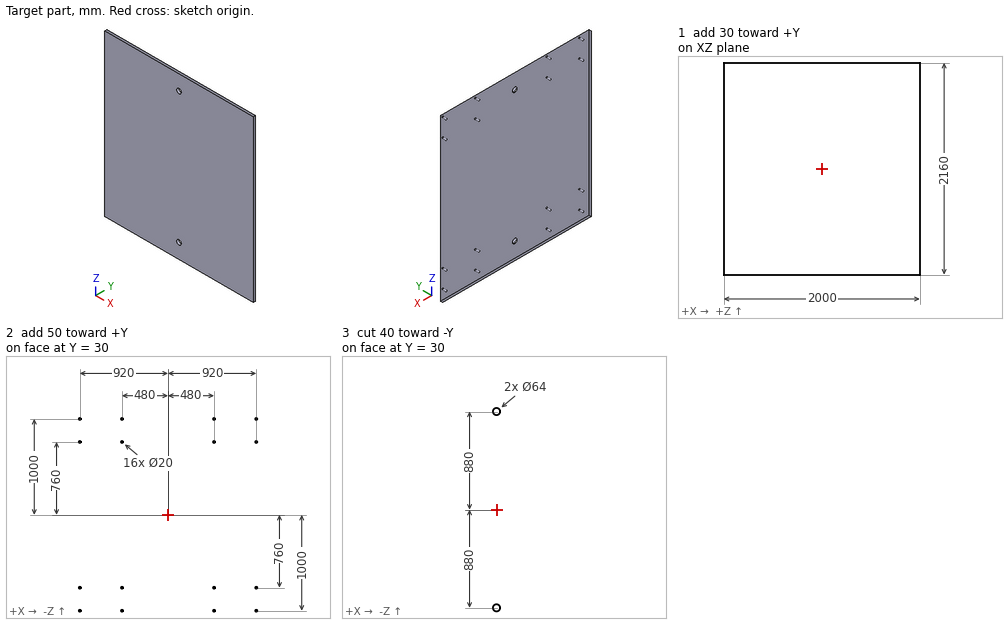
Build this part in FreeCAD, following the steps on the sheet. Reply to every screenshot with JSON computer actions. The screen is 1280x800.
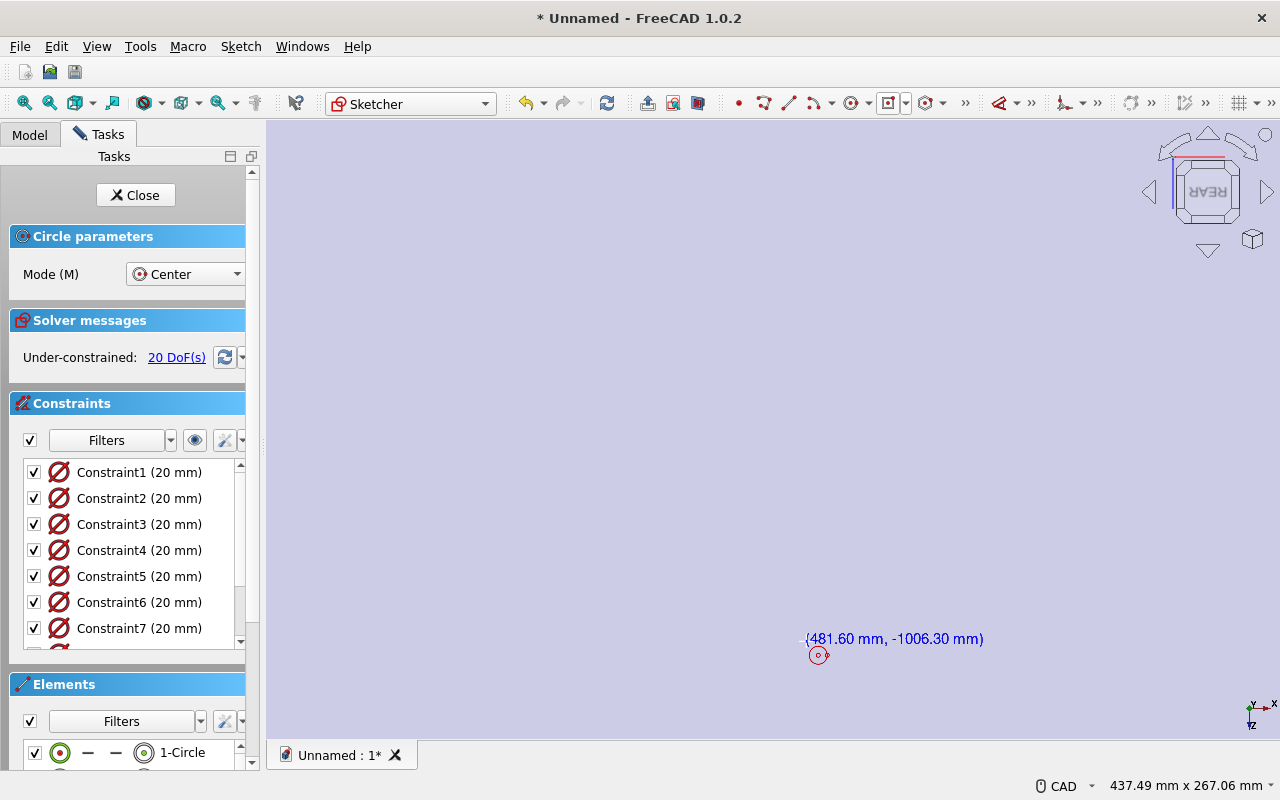
{"action": "scroll", "coordinate": [806, 641], "scroll_direction": "down", "scroll_amount": 12}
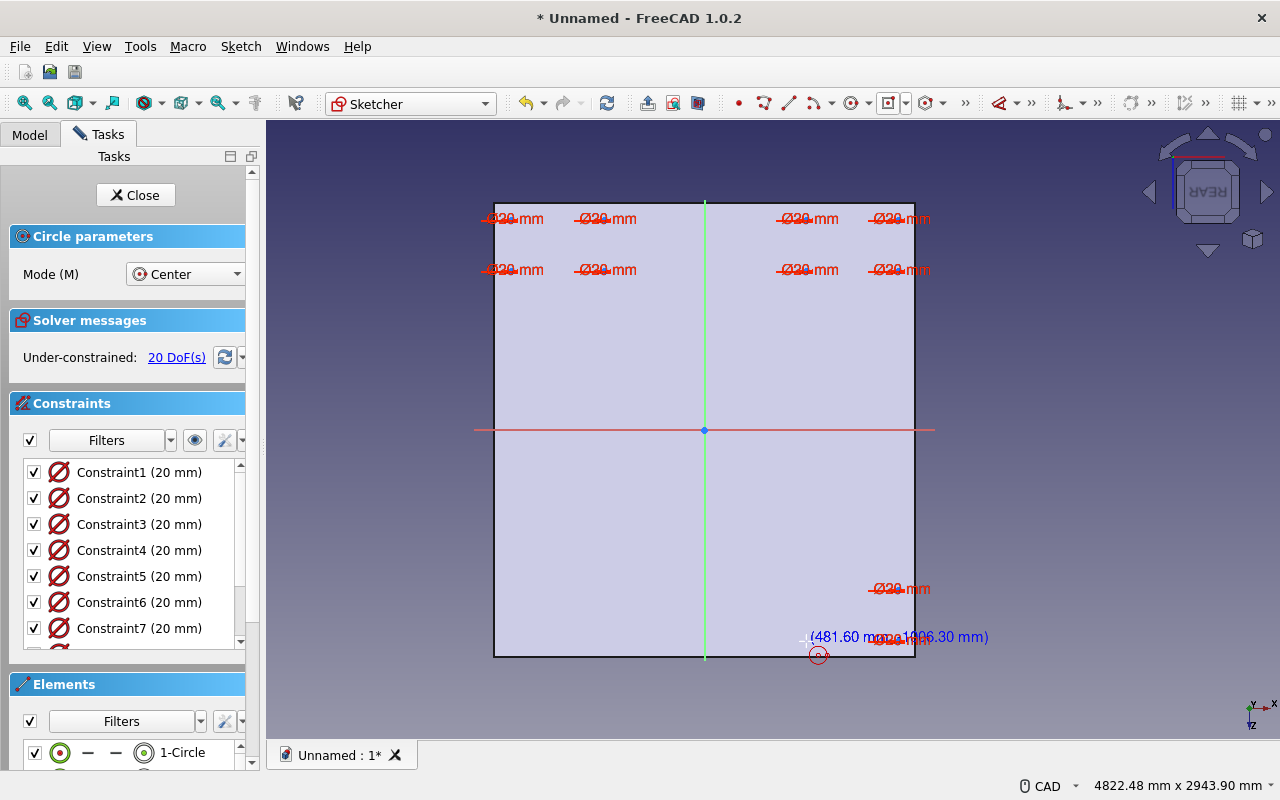
{"action": "left_click", "coordinate": [806, 641]}
{"action": "mouse_move", "coordinate": [807, 639]}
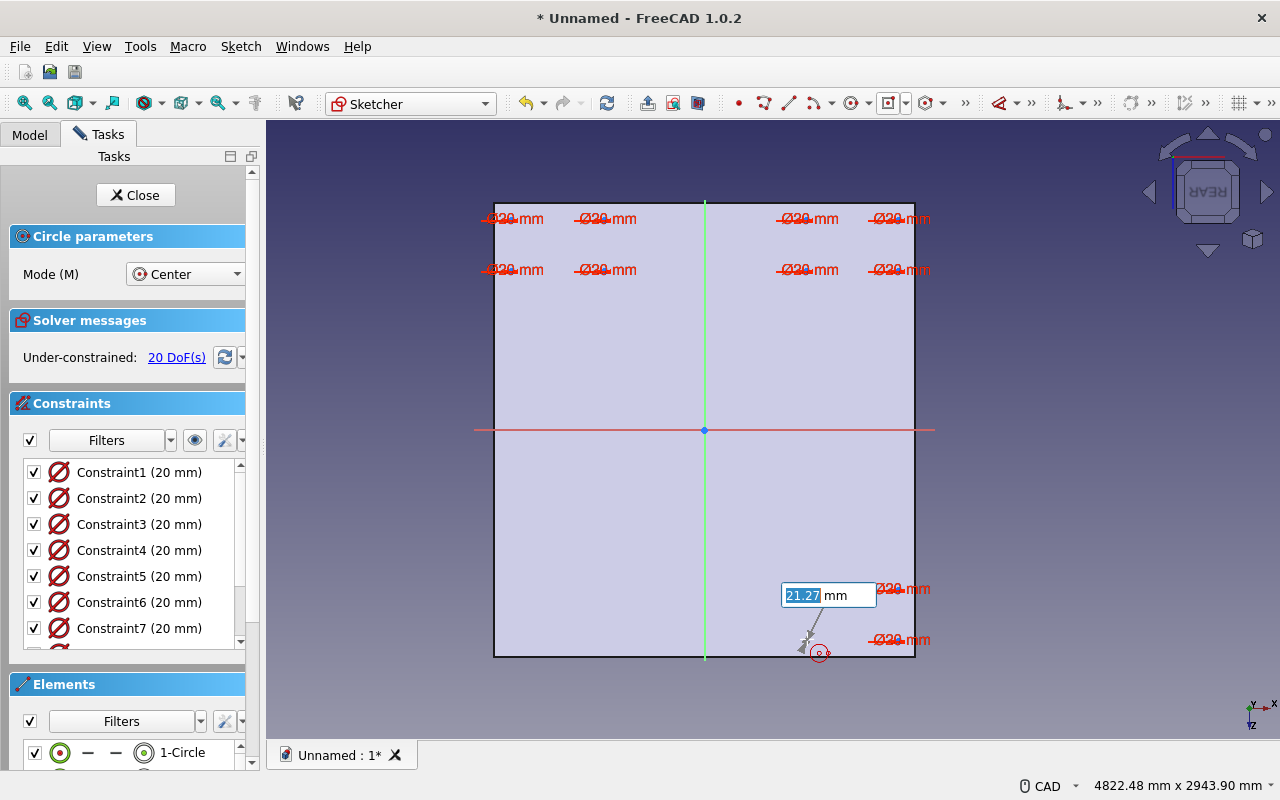
{"action": "type", "text": "20"}
{"action": "key", "text": "Return"}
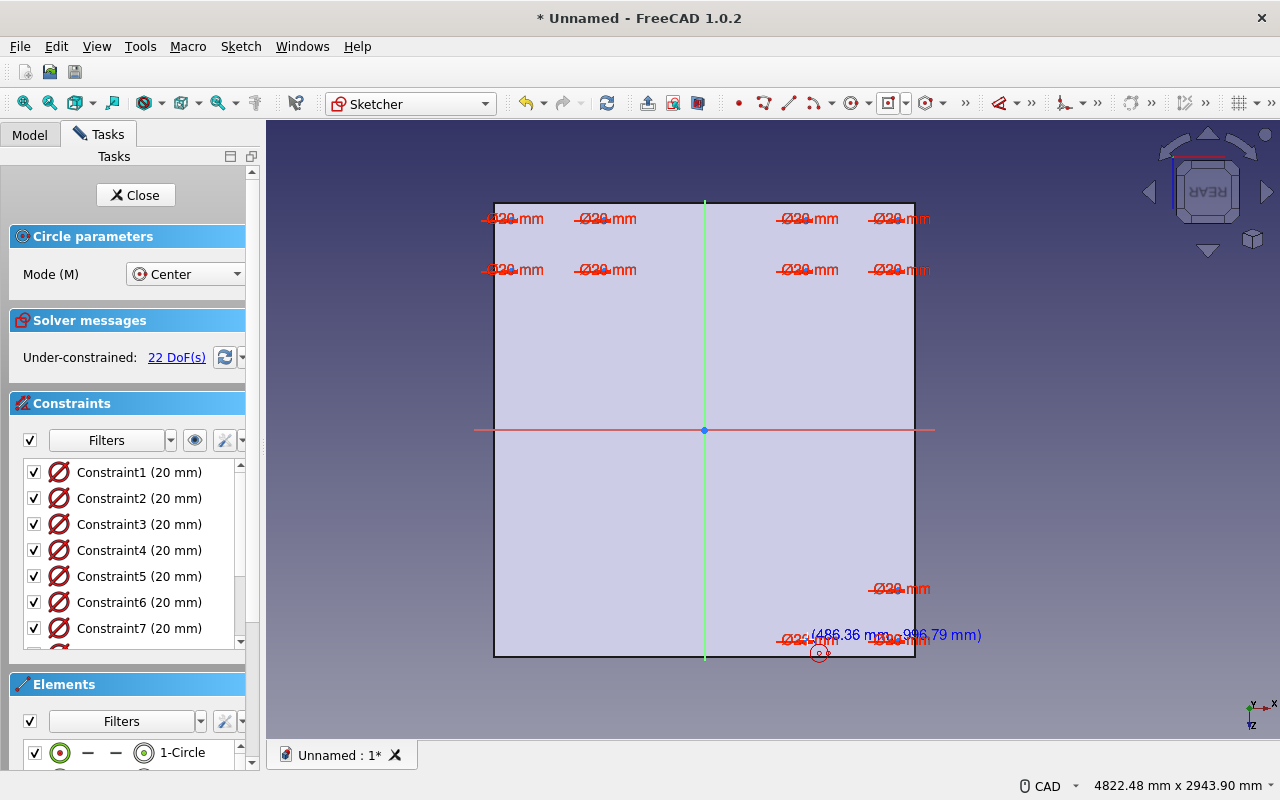
{"action": "scroll", "coordinate": [806, 590], "scroll_direction": "up", "scroll_amount": 12}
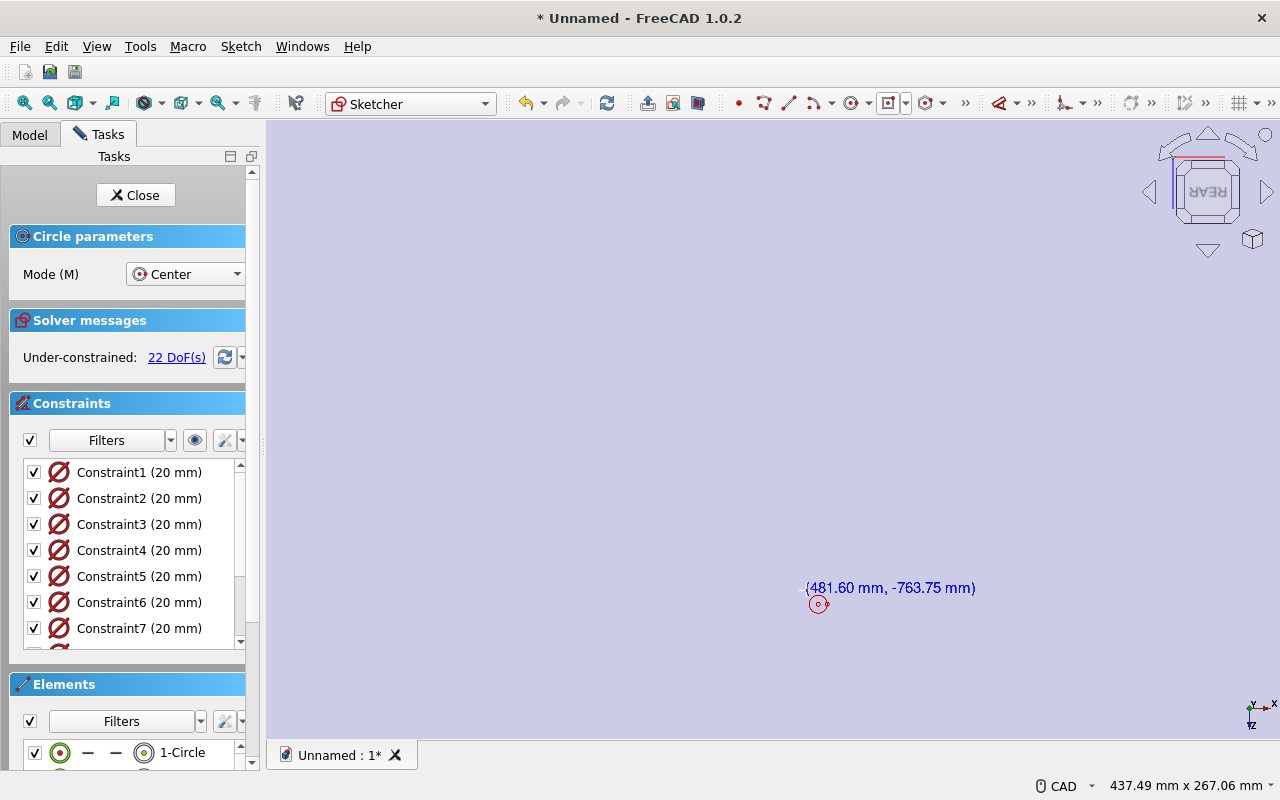
{"action": "scroll", "coordinate": [806, 590], "scroll_direction": "down", "scroll_amount": 12}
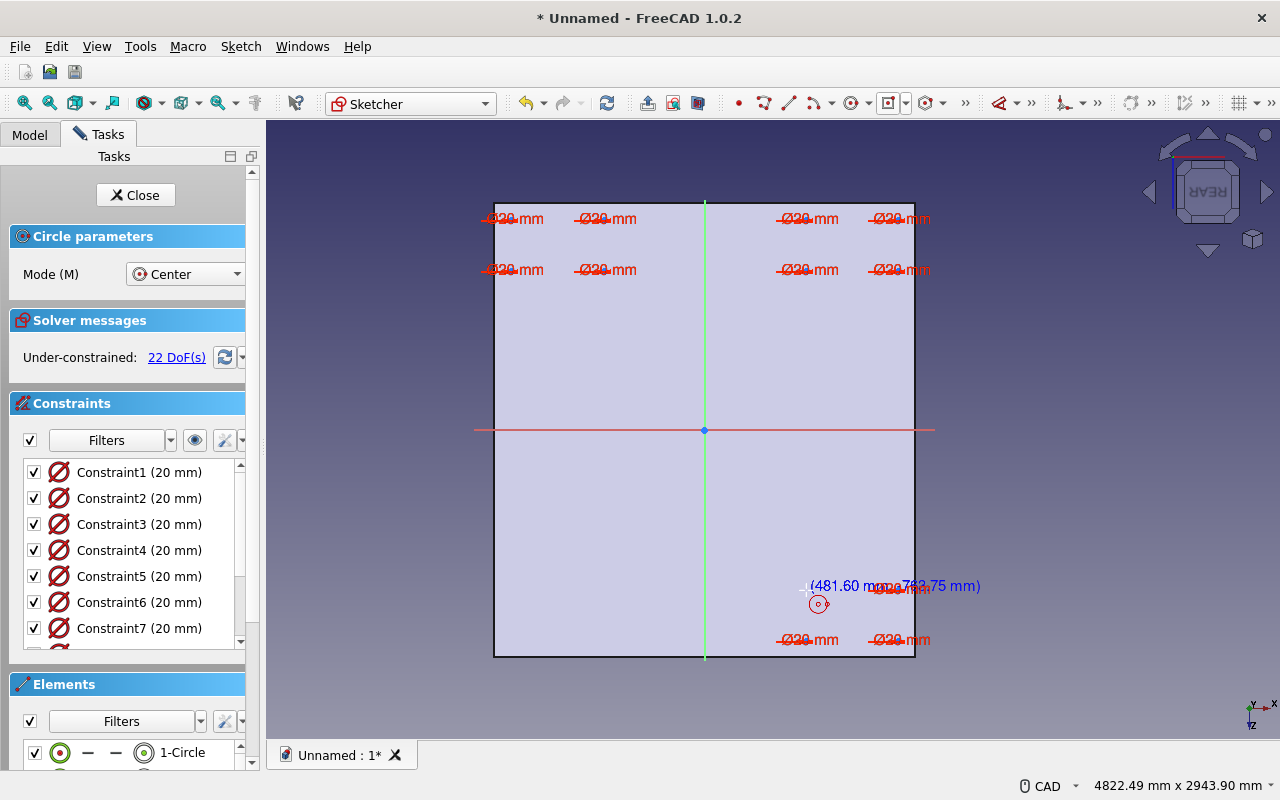
{"action": "left_click", "coordinate": [806, 590]}
{"action": "mouse_move", "coordinate": [807, 589]}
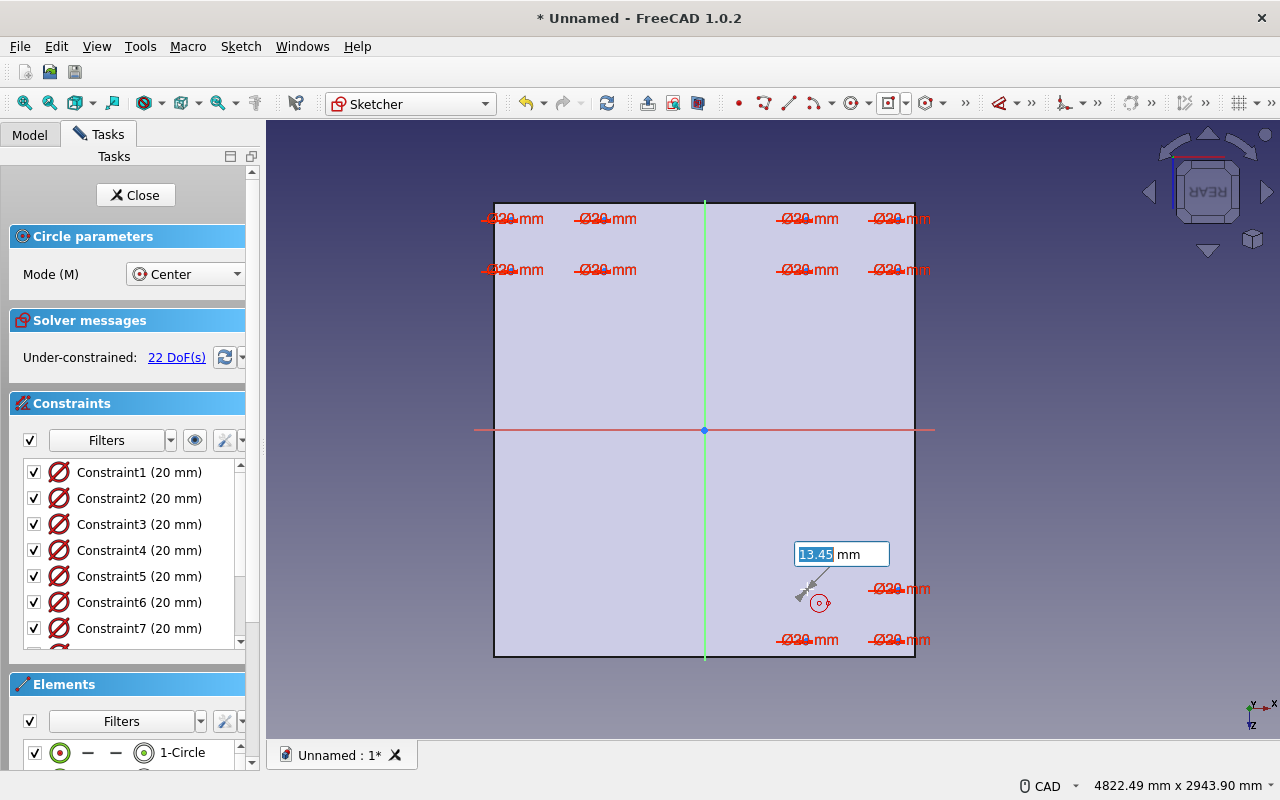
{"action": "type", "text": "20"}
{"action": "key", "text": "Return"}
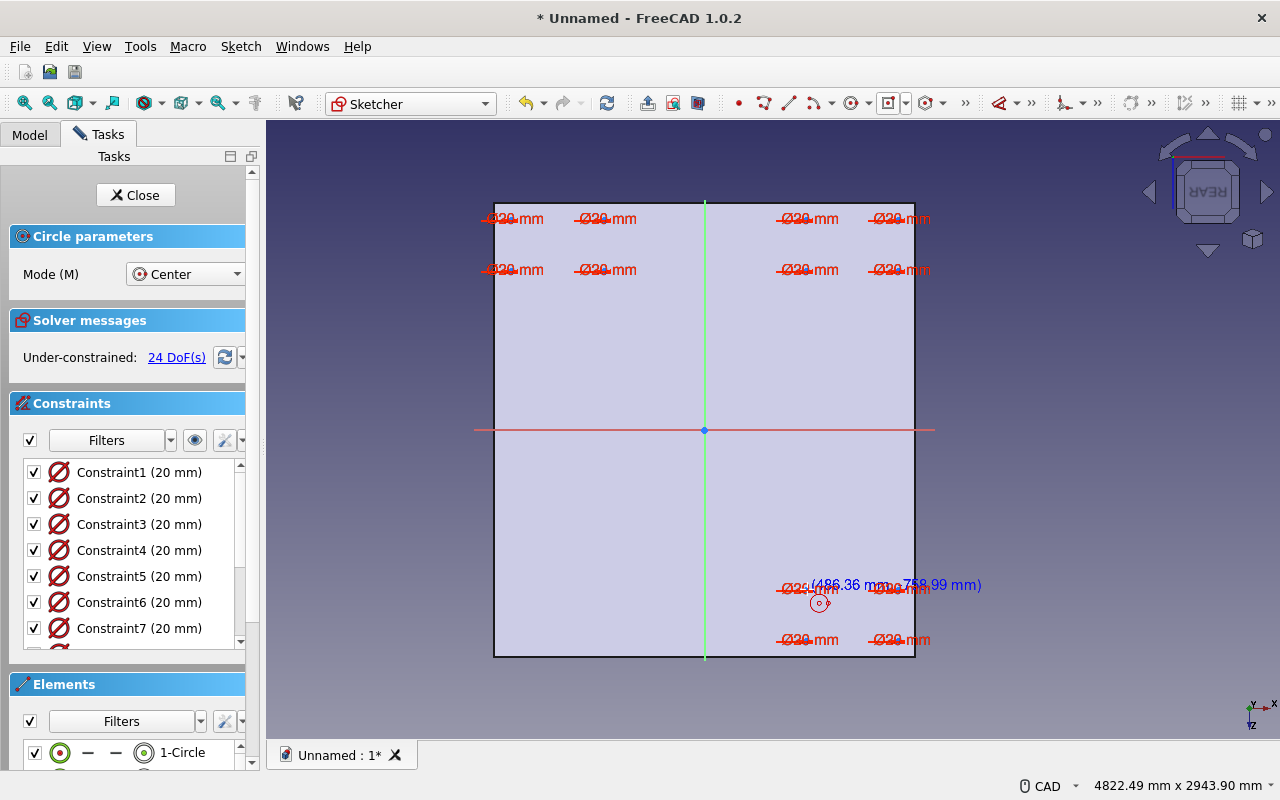
{"action": "scroll", "coordinate": [604, 590], "scroll_direction": "up", "scroll_amount": 12}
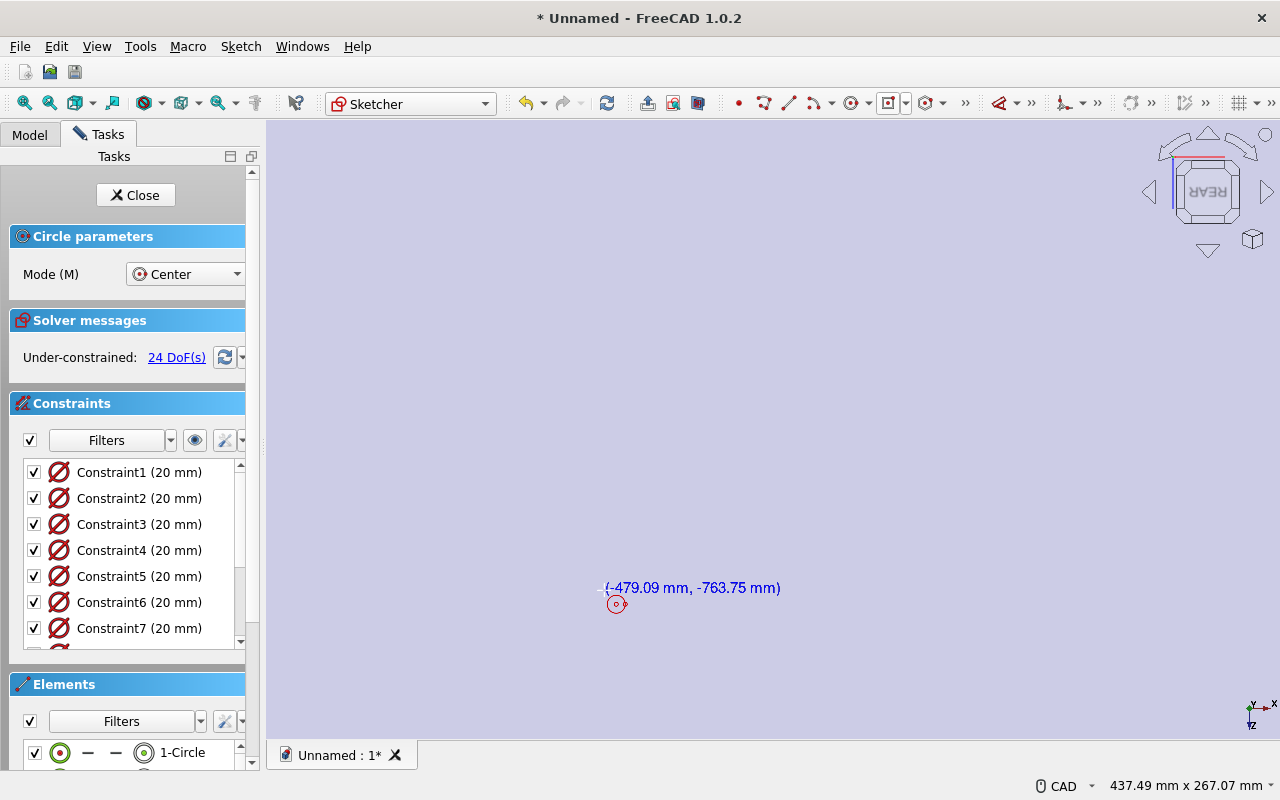
{"action": "scroll", "coordinate": [604, 590], "scroll_direction": "down", "scroll_amount": 12}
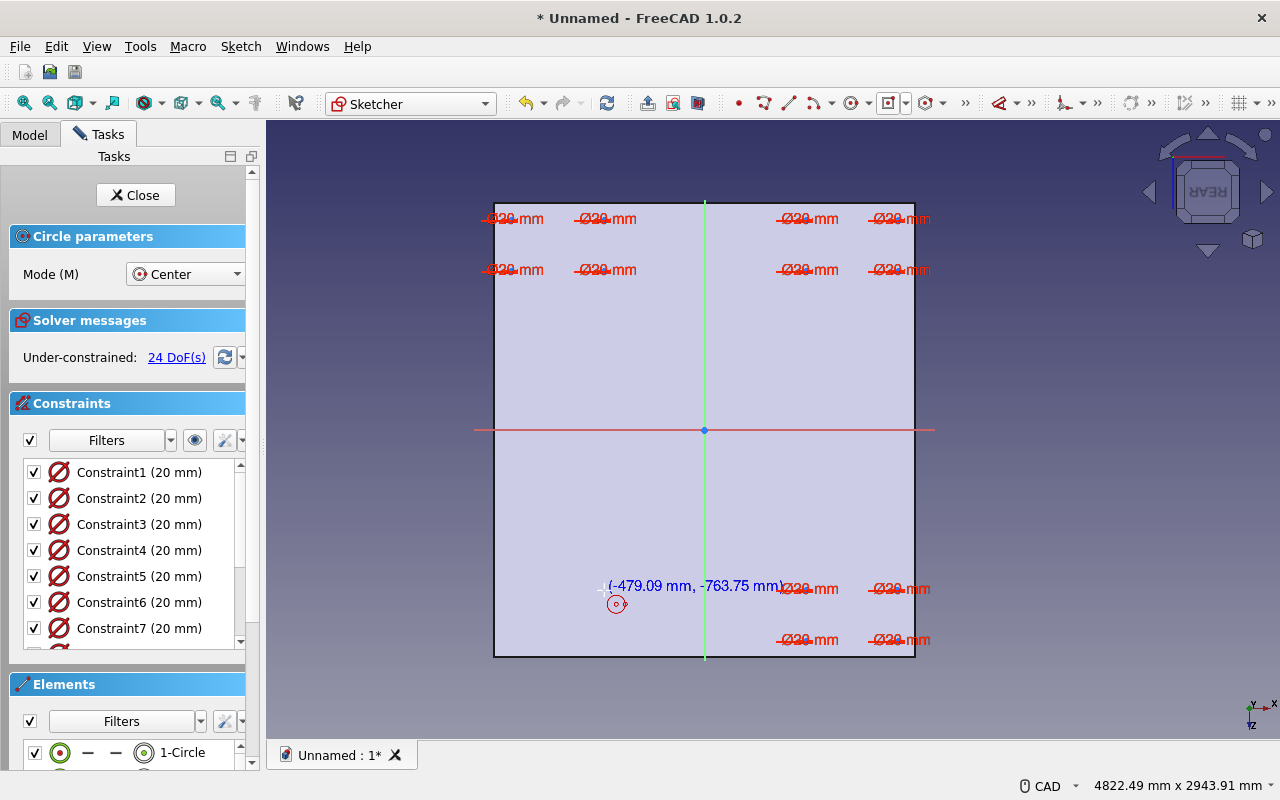
{"action": "left_click", "coordinate": [604, 590]}
{"action": "mouse_move", "coordinate": [605, 589]}